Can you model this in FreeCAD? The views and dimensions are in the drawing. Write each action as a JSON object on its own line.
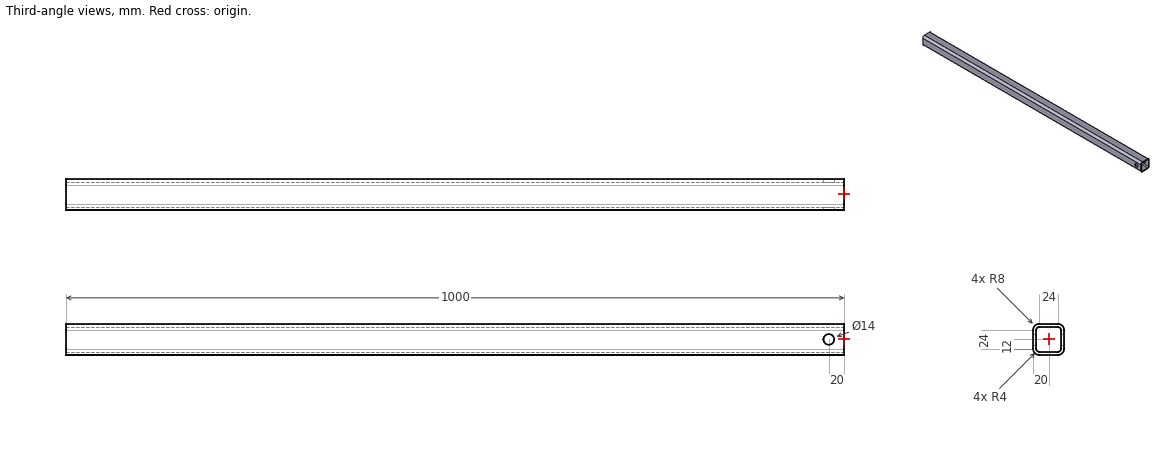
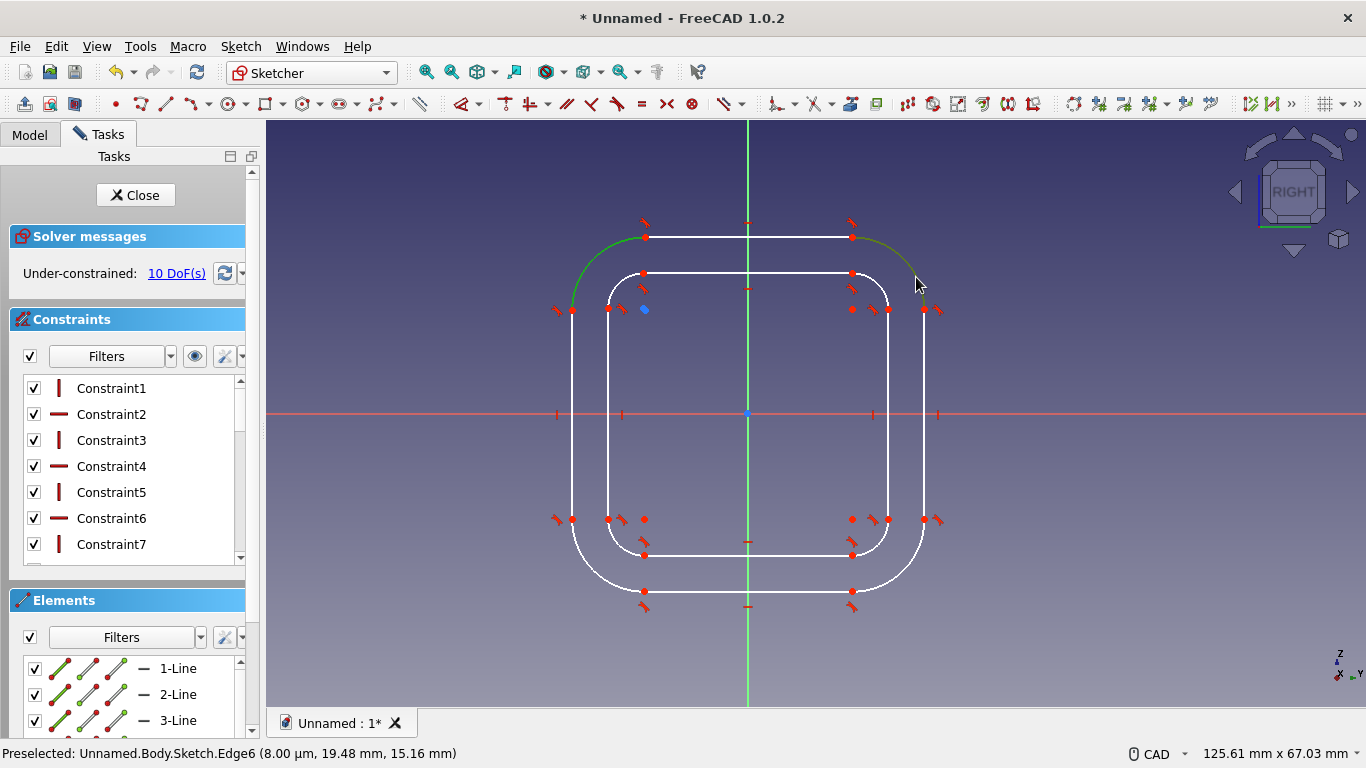
{"action": "left_click", "coordinate": [885, 584]}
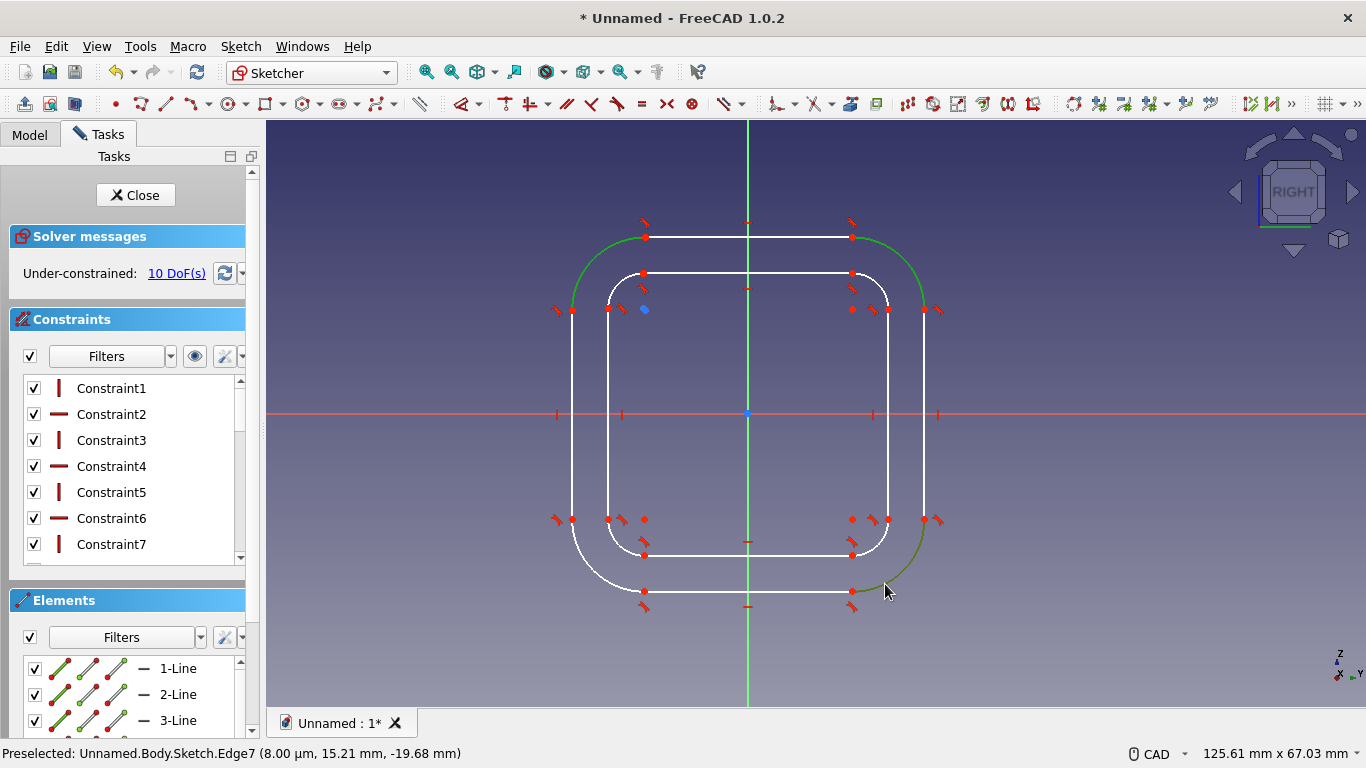
{"action": "left_click", "coordinate": [580, 552]}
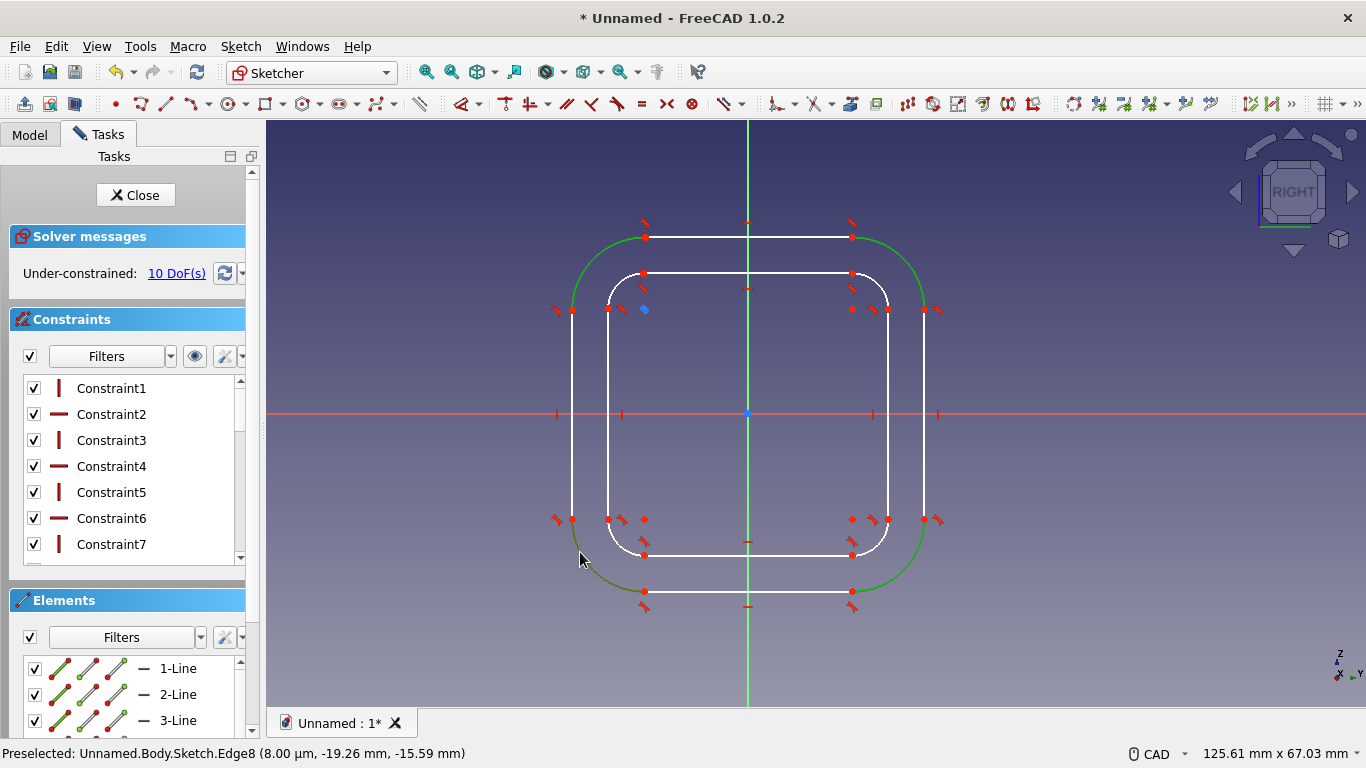
{"action": "left_click", "coordinate": [642, 104]}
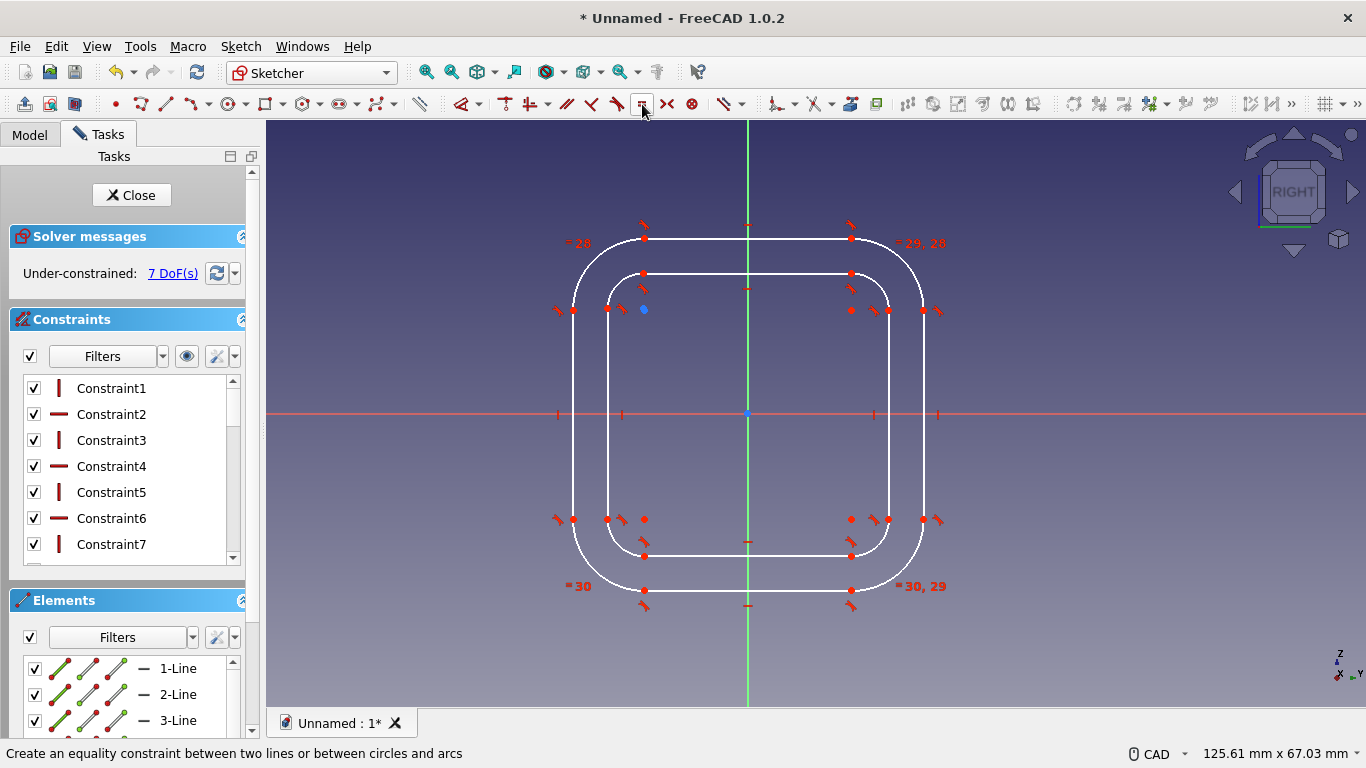
{"action": "left_click", "coordinate": [612, 536]}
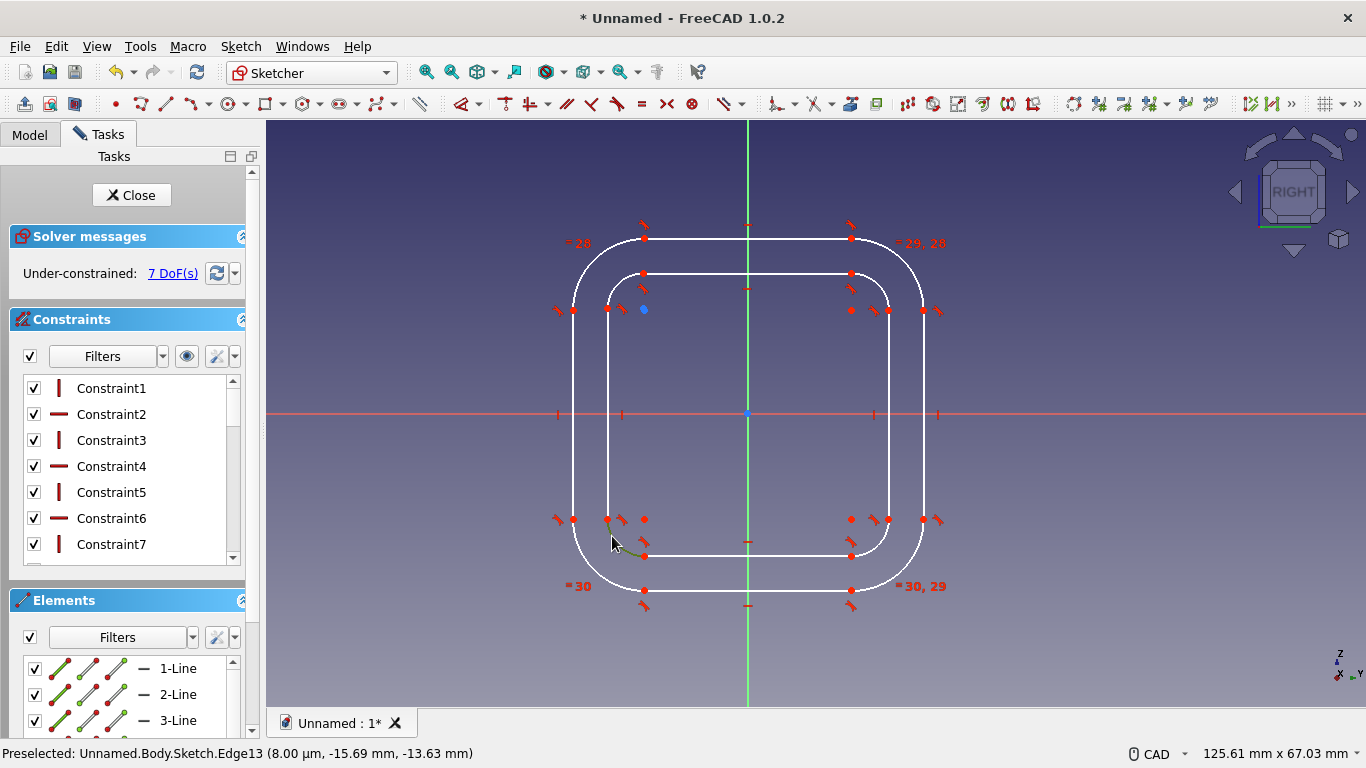
{"action": "left_click", "coordinate": [627, 277]}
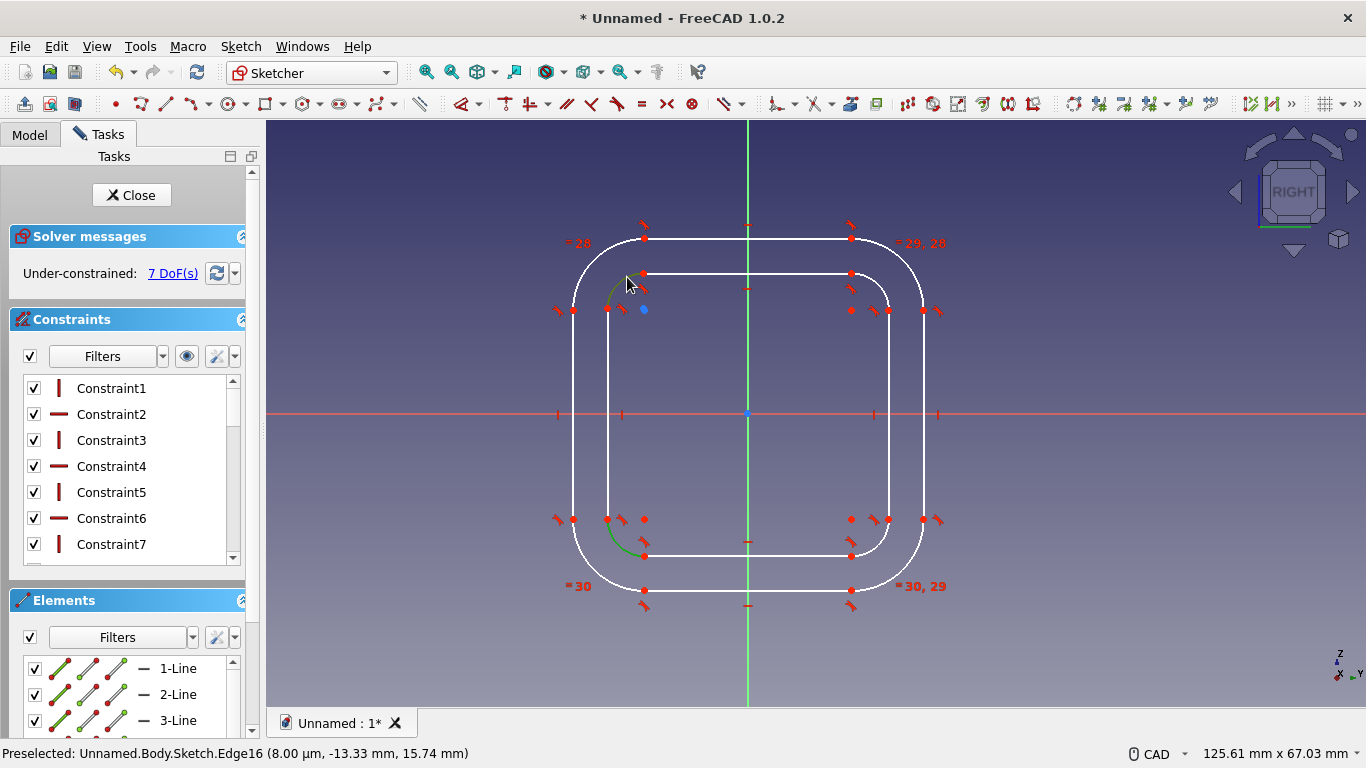
{"action": "left_click", "coordinate": [642, 104]}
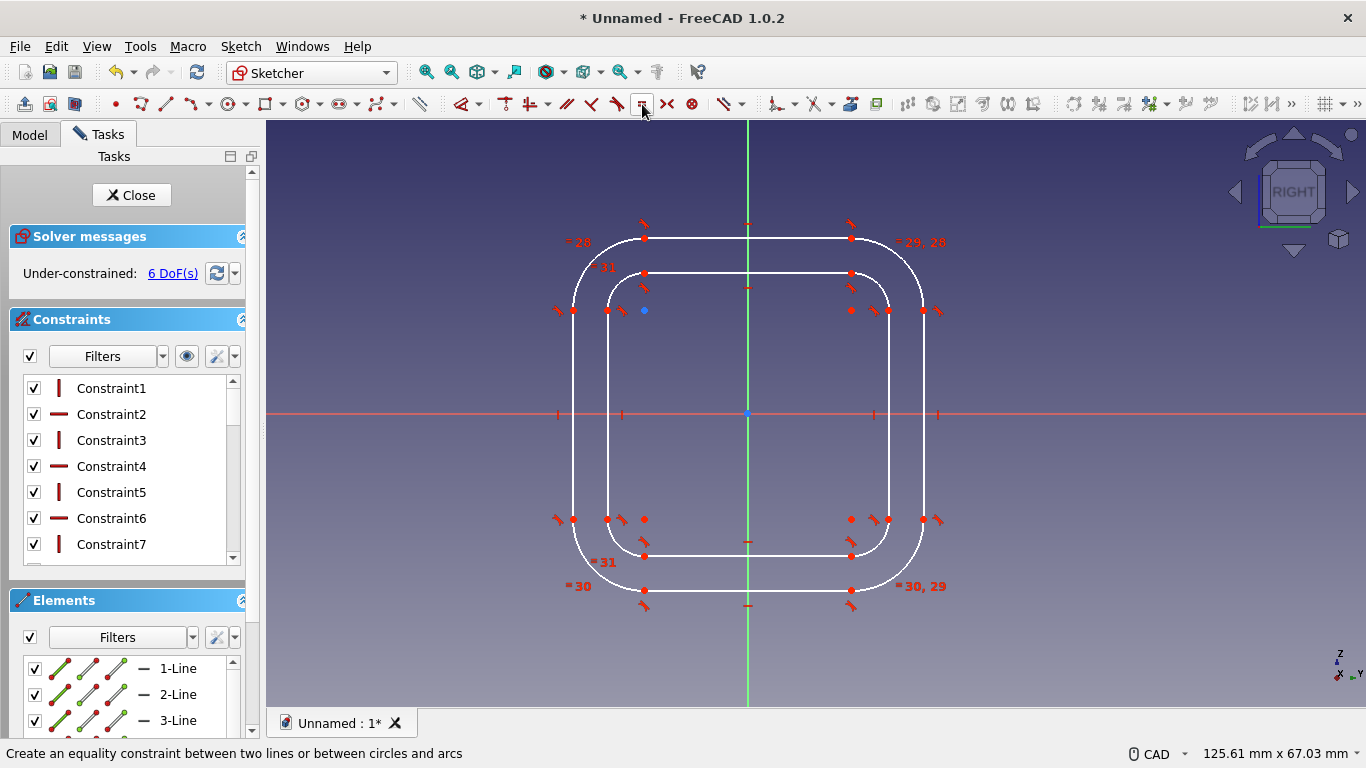
{"action": "left_click", "coordinate": [612, 246]}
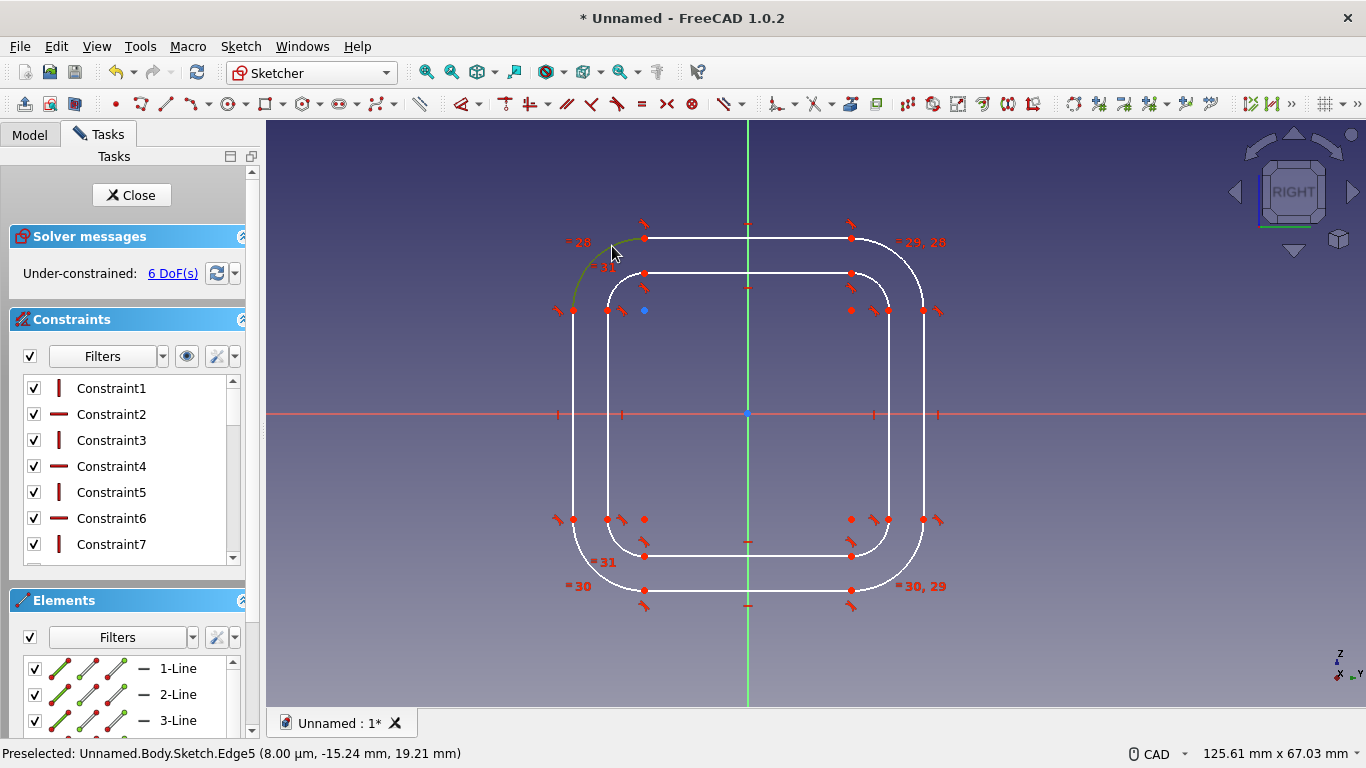
{"action": "left_click", "coordinate": [478, 104]}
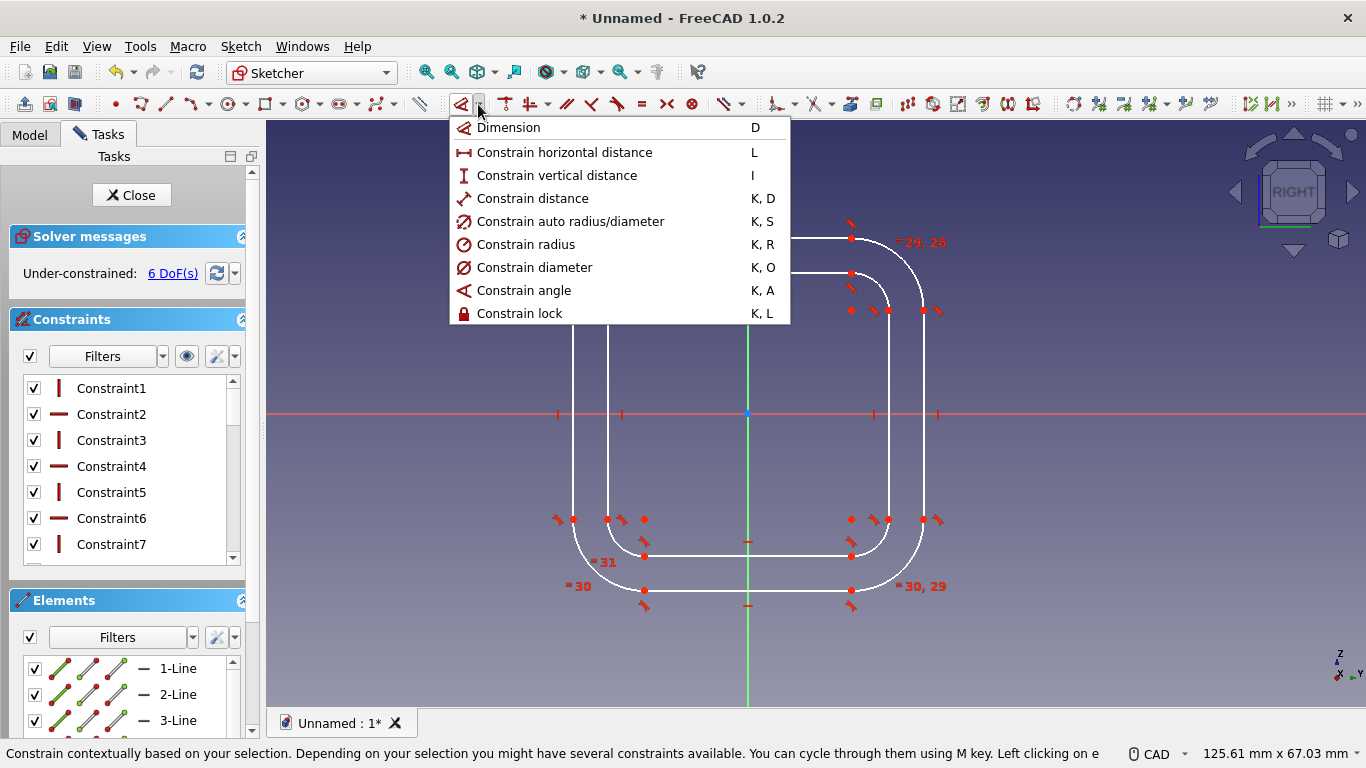
{"action": "left_click", "coordinate": [620, 244]}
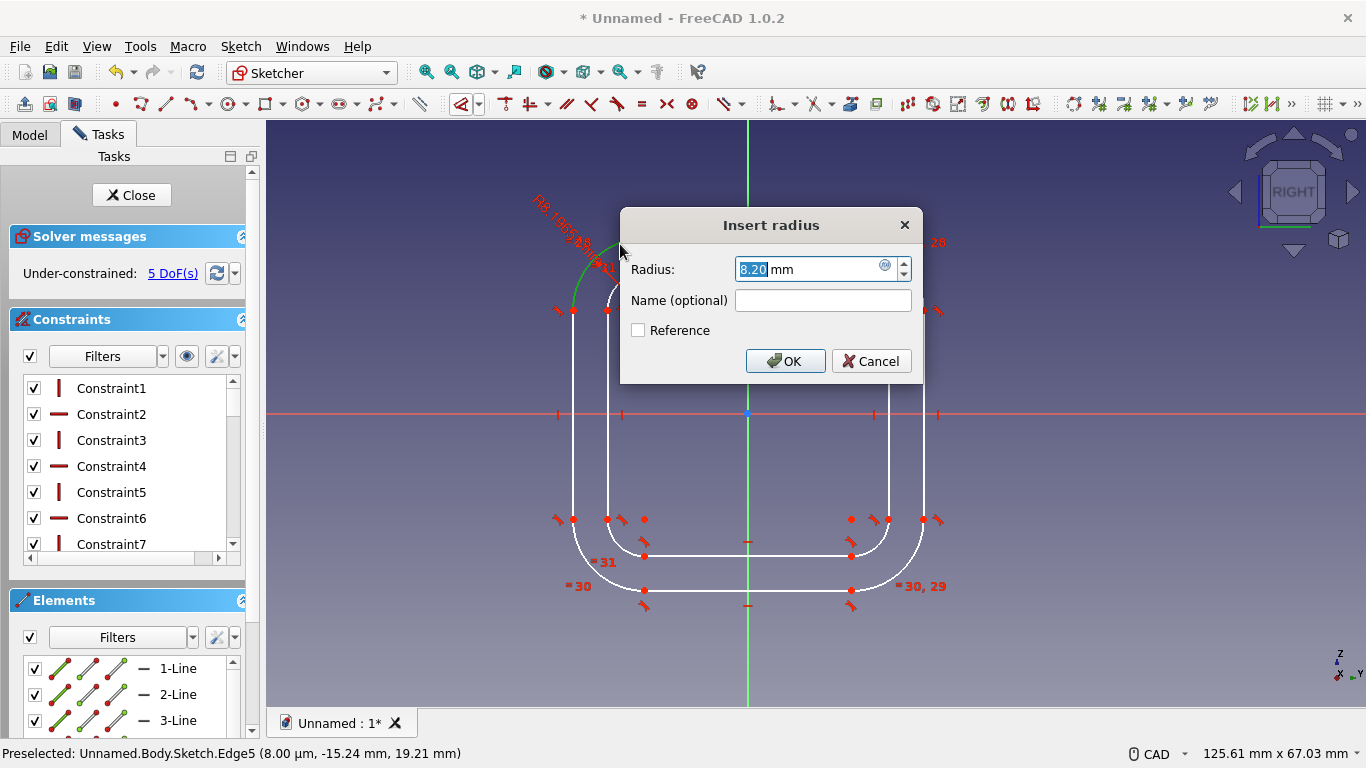
{"action": "type", "text": "8"}
{"action": "key", "text": "Return"}